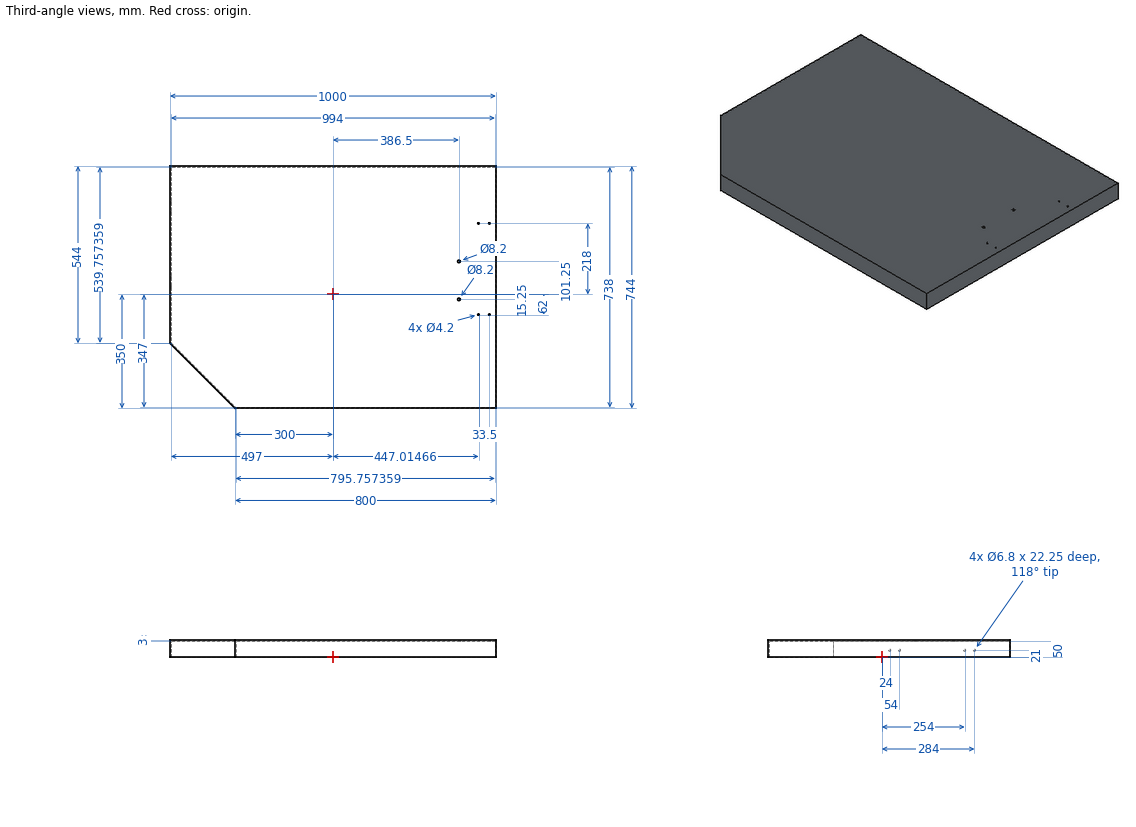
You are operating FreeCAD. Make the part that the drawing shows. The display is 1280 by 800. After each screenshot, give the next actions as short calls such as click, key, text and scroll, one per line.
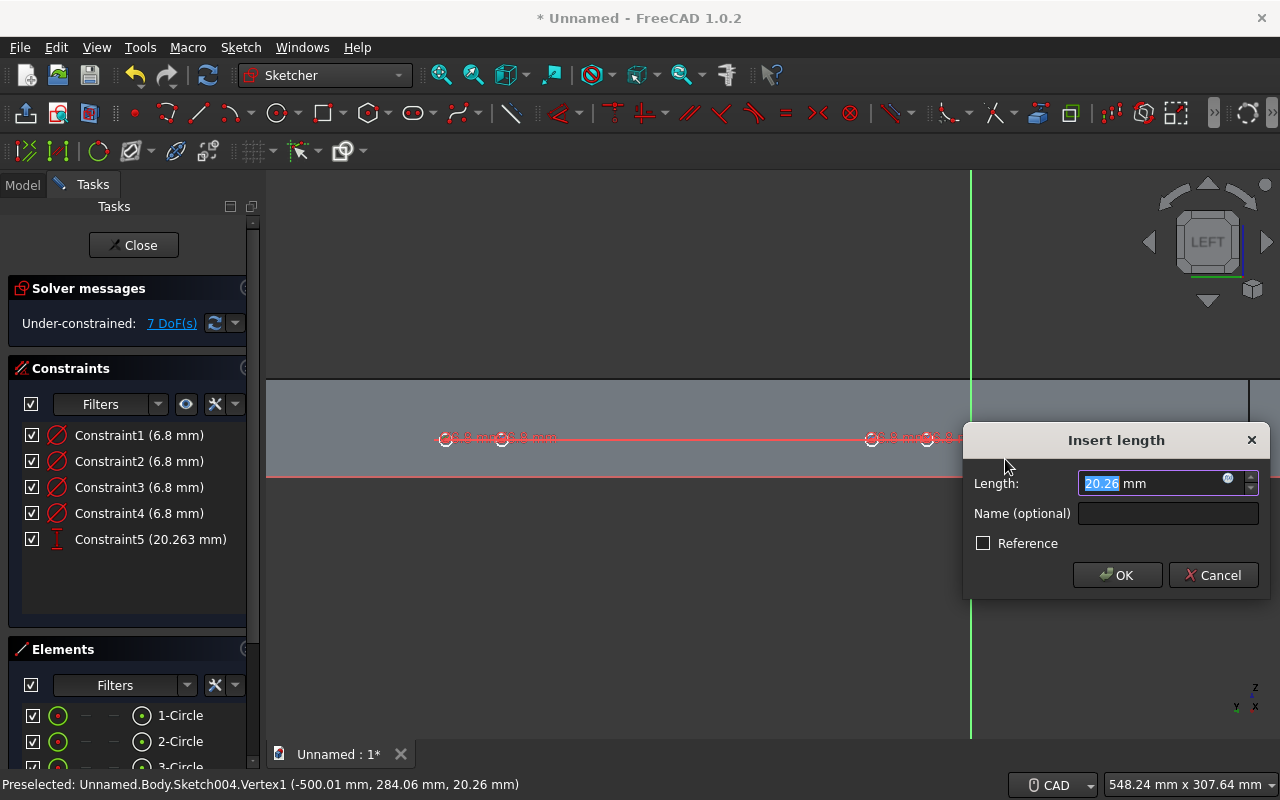
text(21)
key(Return)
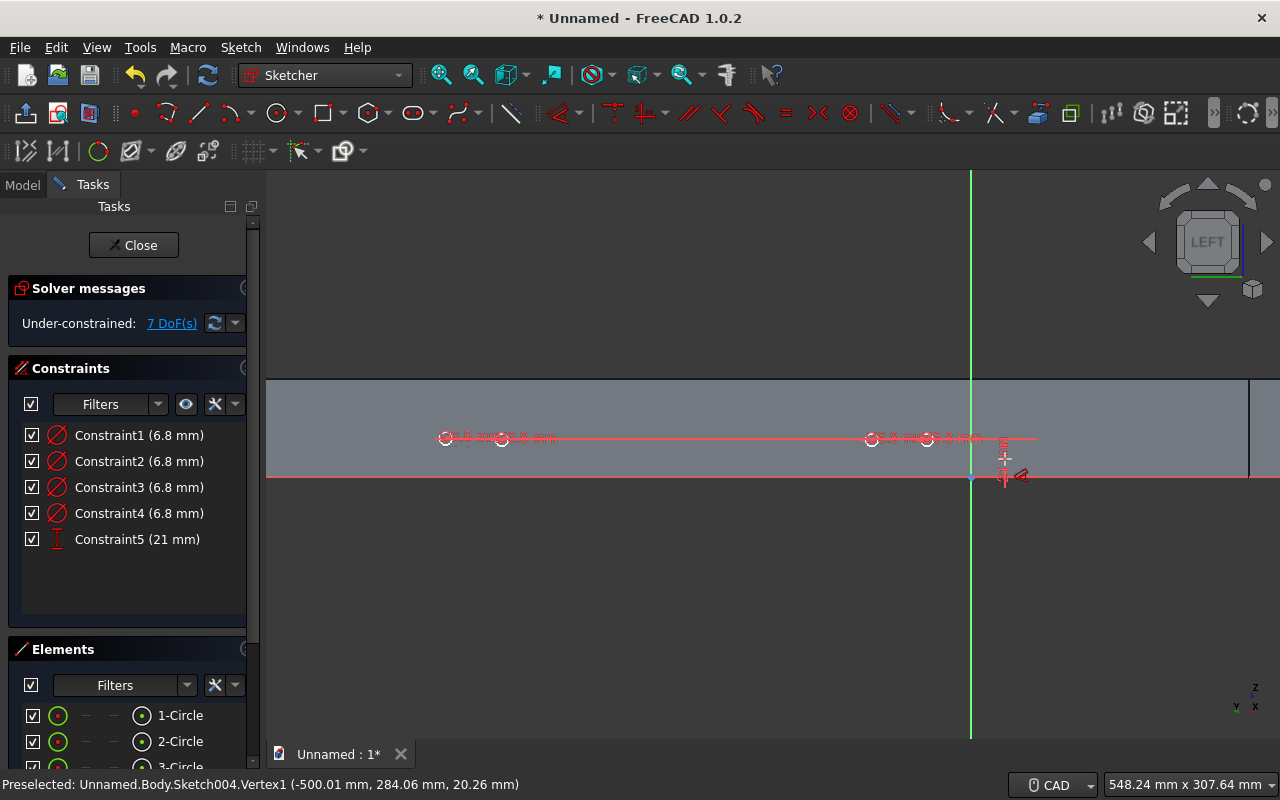
click(502, 440)
click(468, 459)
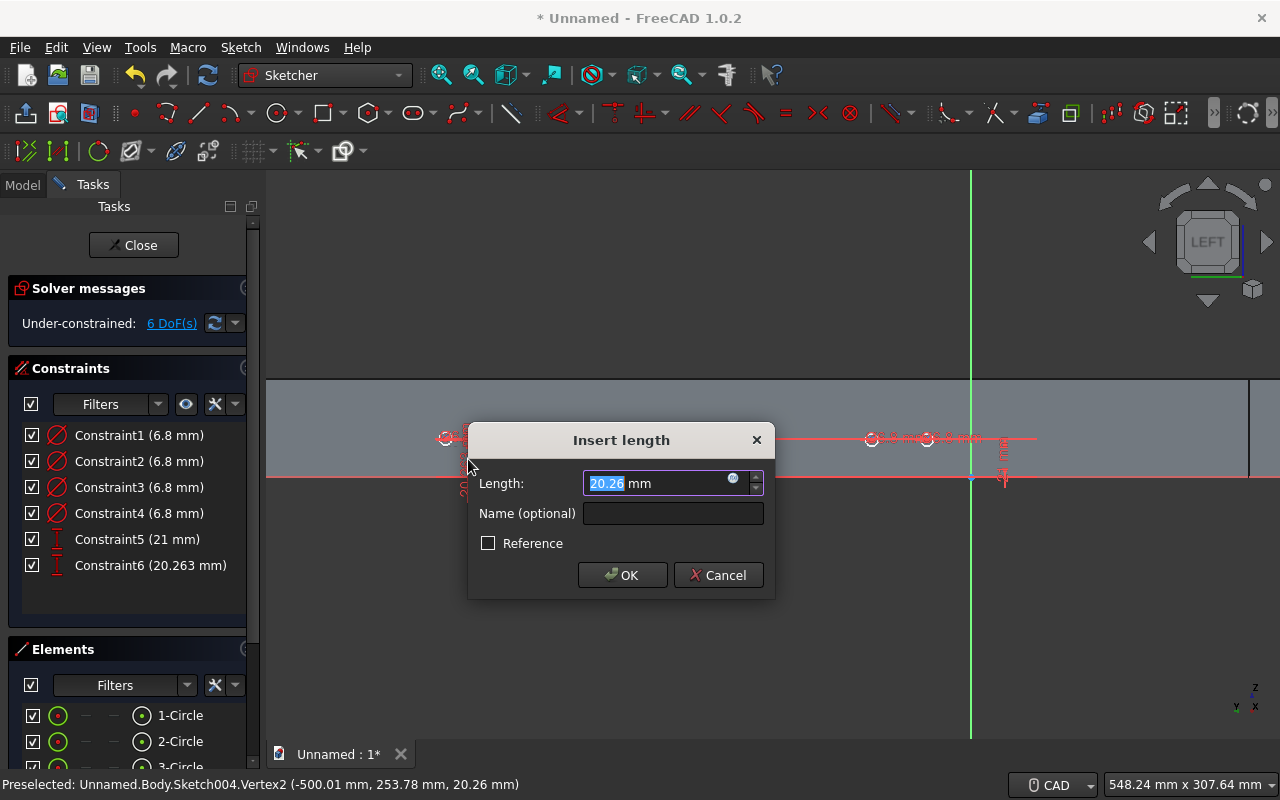
text(21)
key(Return)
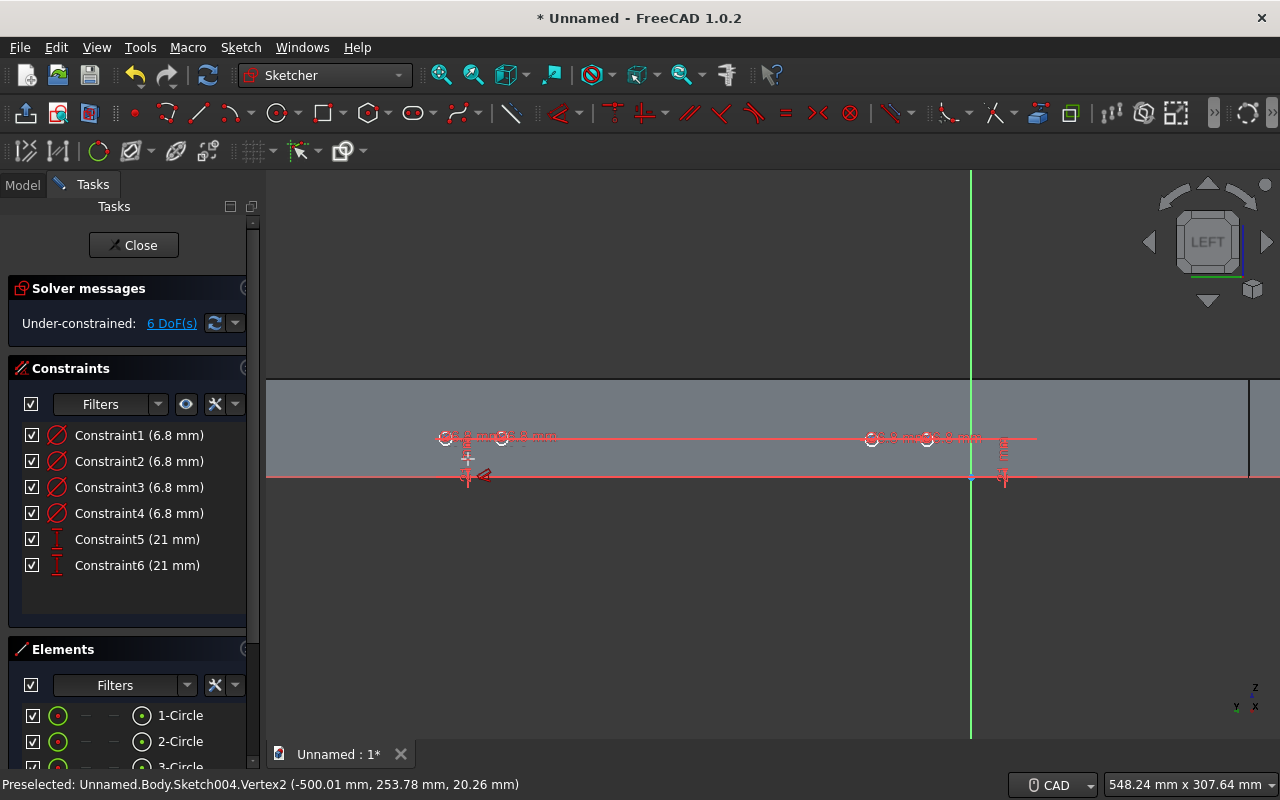
click(872, 440)
click(921, 511)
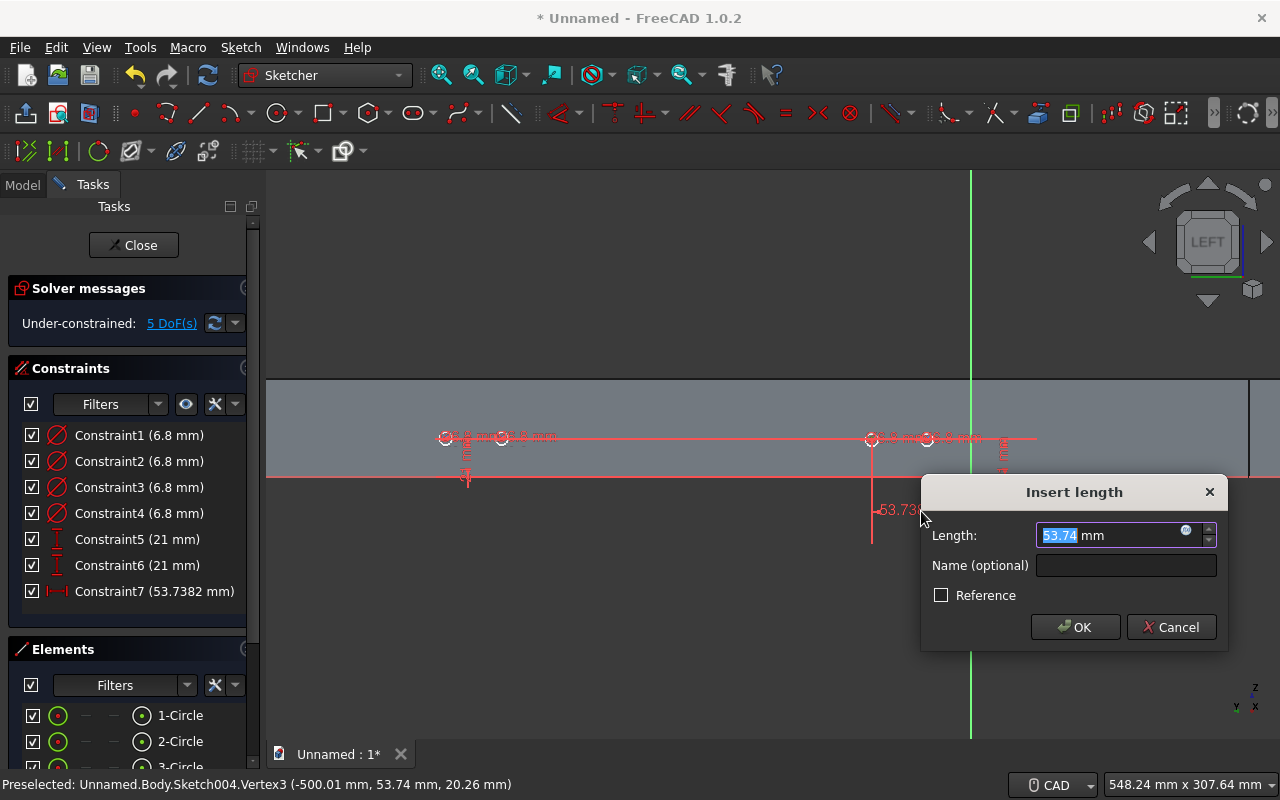
text(54)
key(Return)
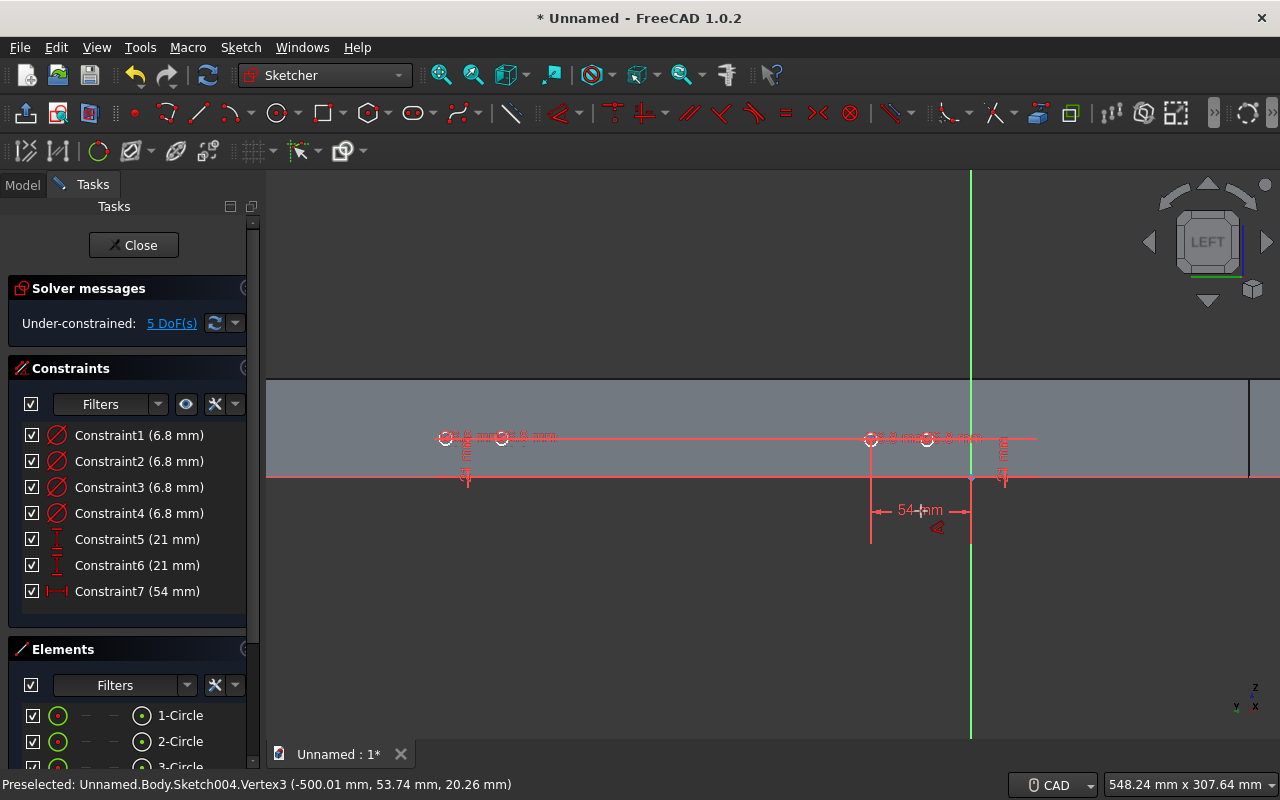
click(871, 440)
click(837, 459)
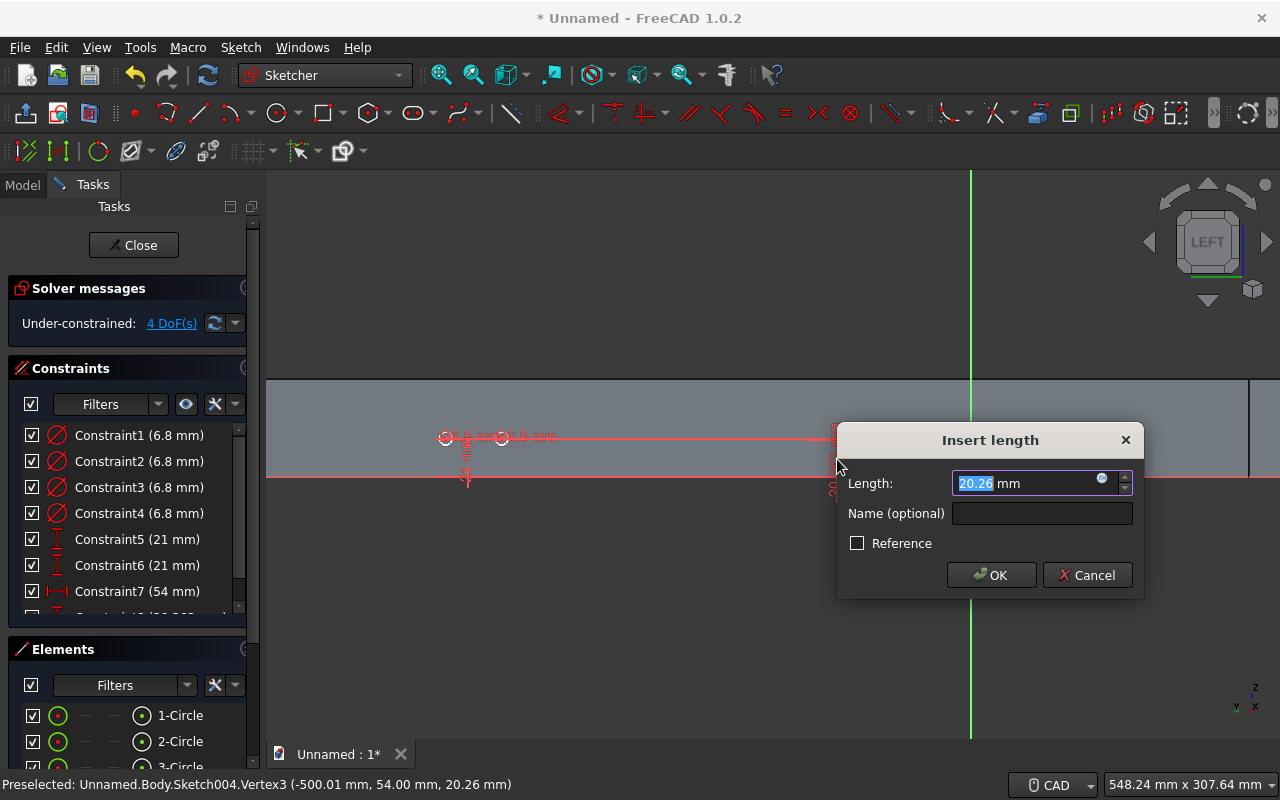
text(21)
key(Return)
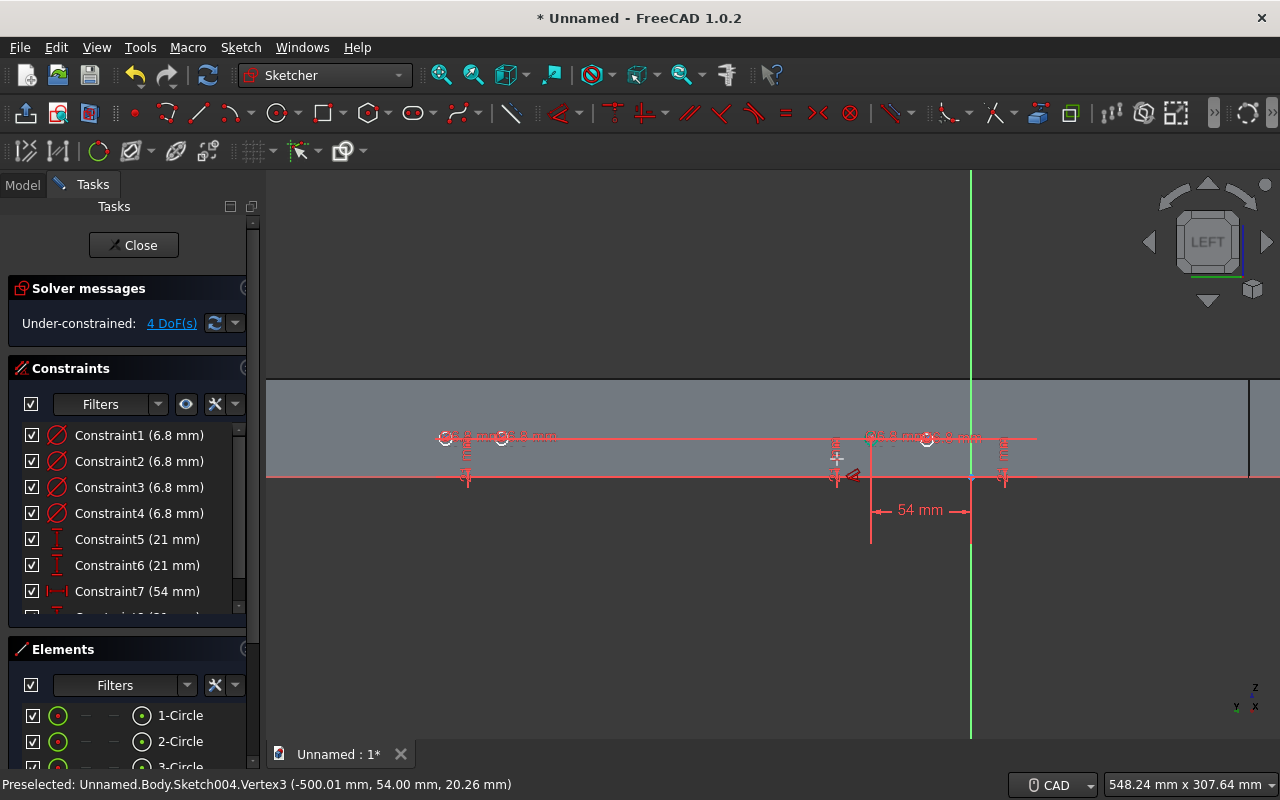
click(927, 440)
click(949, 406)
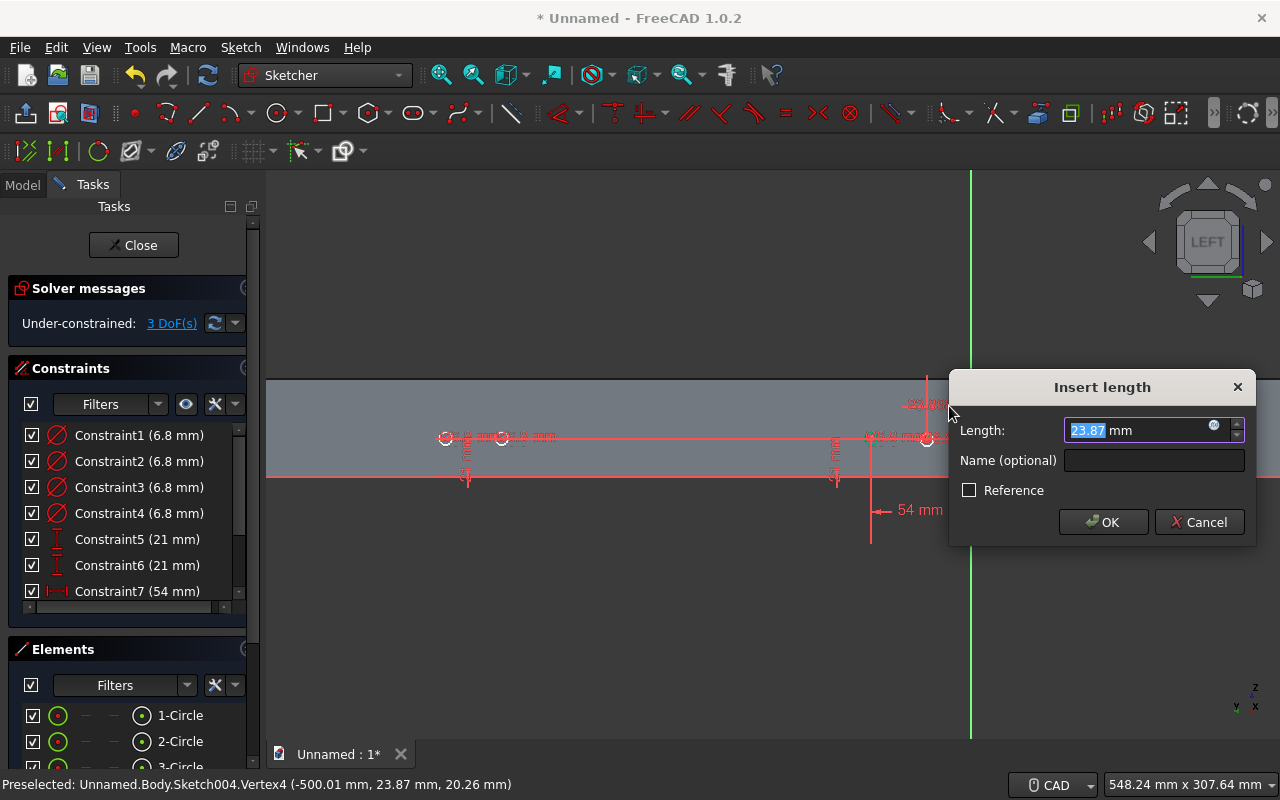
text(24)
key(Return)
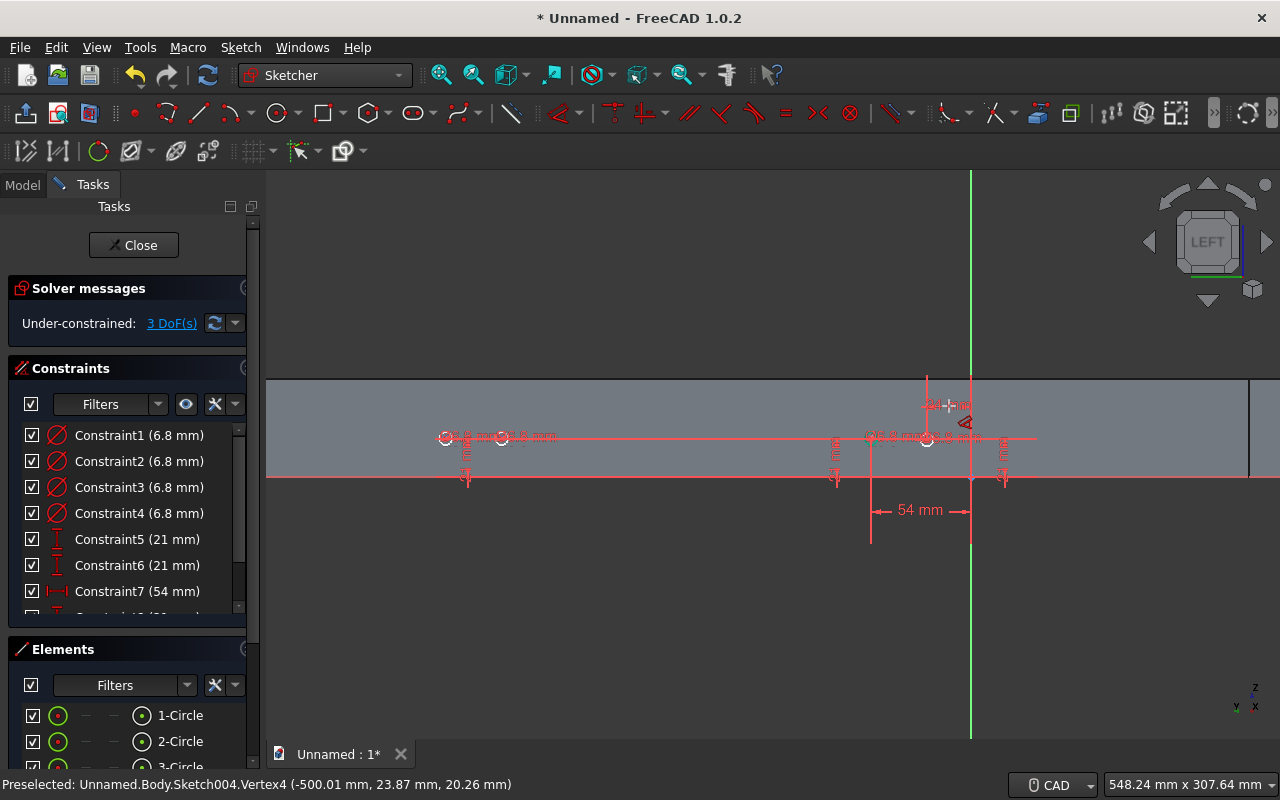
click(927, 440)
click(1077, 459)